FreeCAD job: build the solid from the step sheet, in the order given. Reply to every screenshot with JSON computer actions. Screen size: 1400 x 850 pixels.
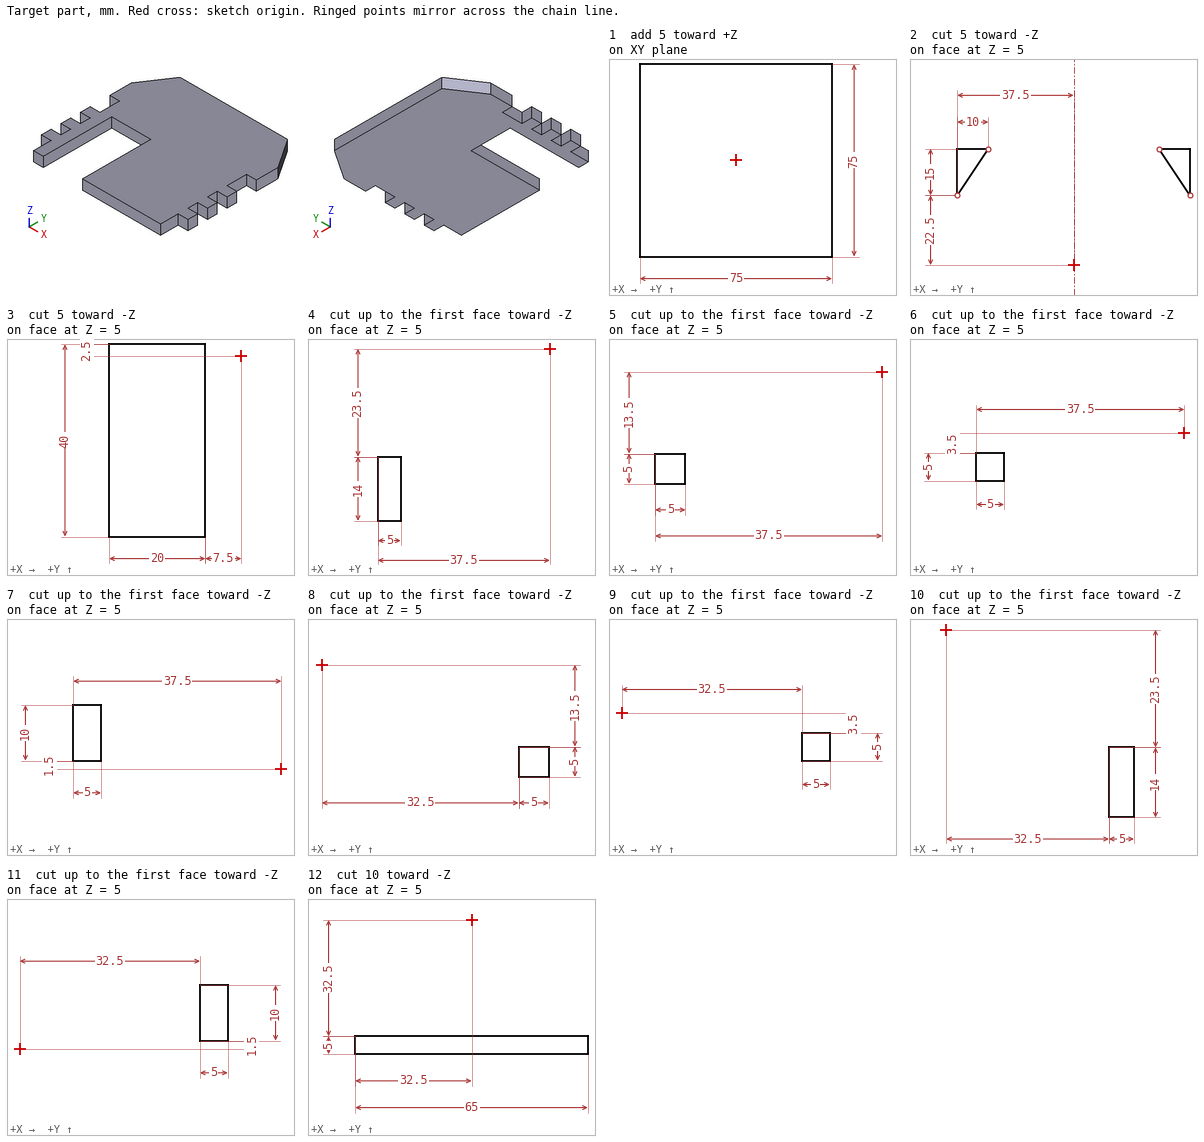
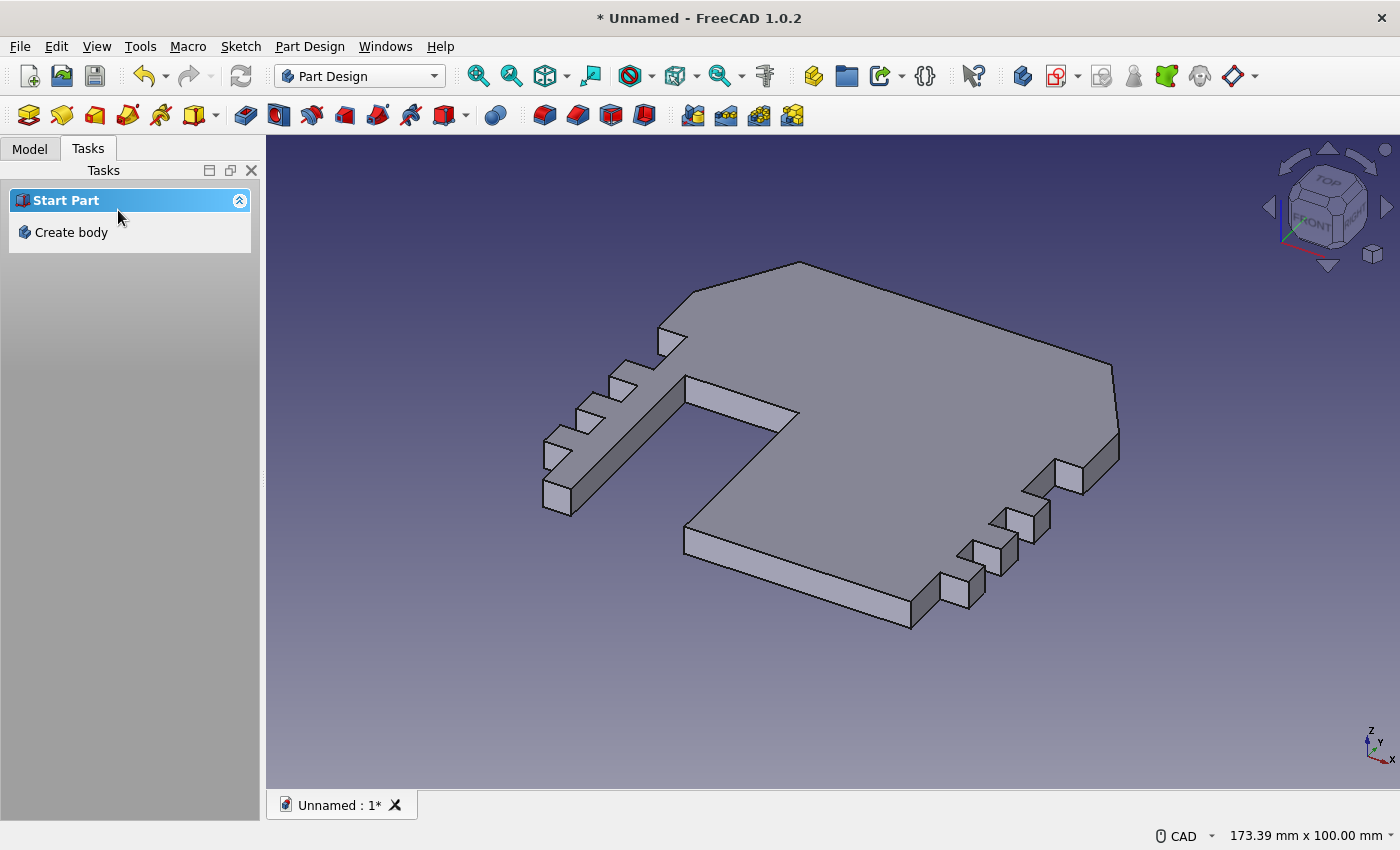
{"action": "key", "text": "0"}